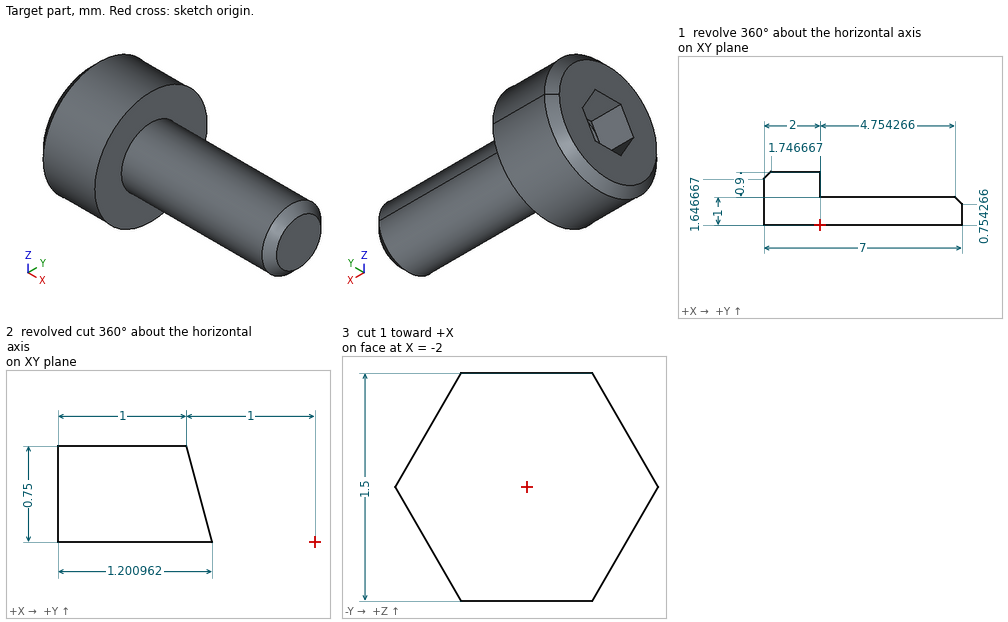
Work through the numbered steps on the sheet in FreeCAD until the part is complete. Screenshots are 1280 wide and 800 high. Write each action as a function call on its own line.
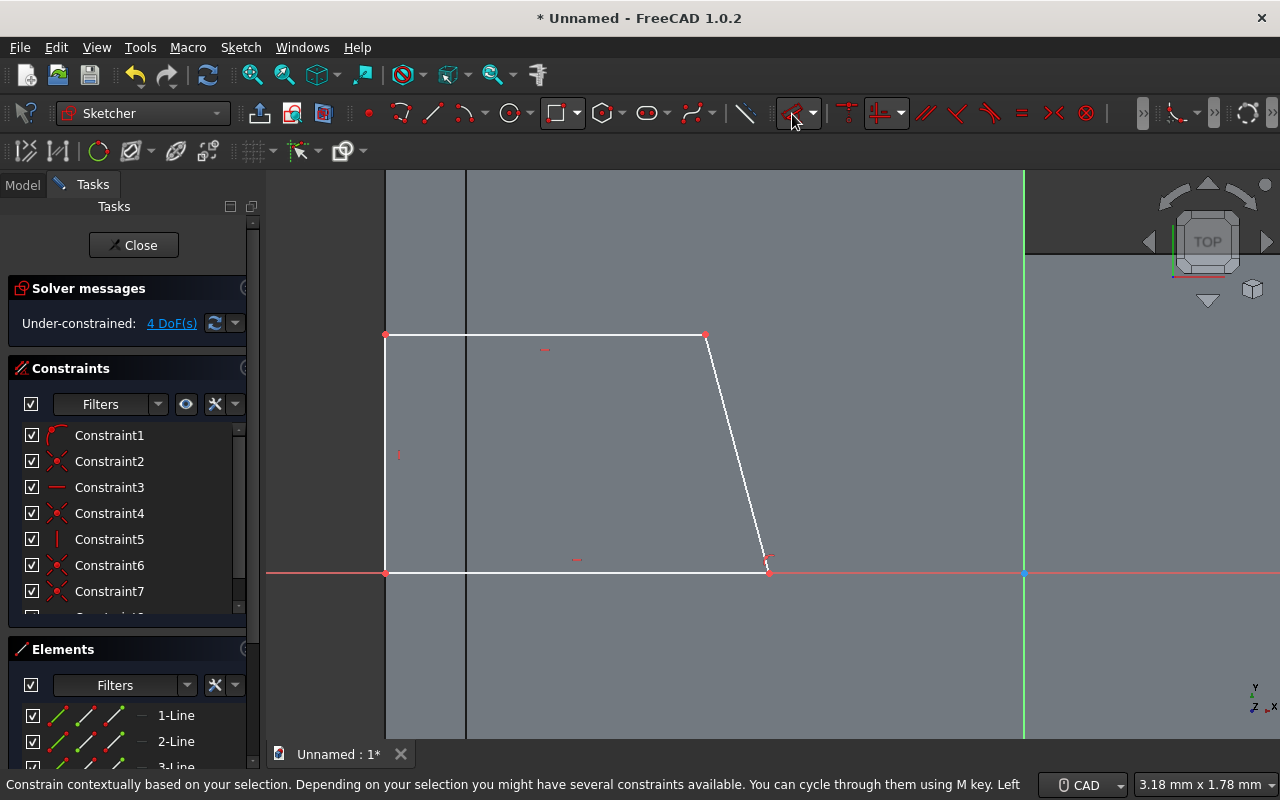
click(609, 335)
click(545, 301)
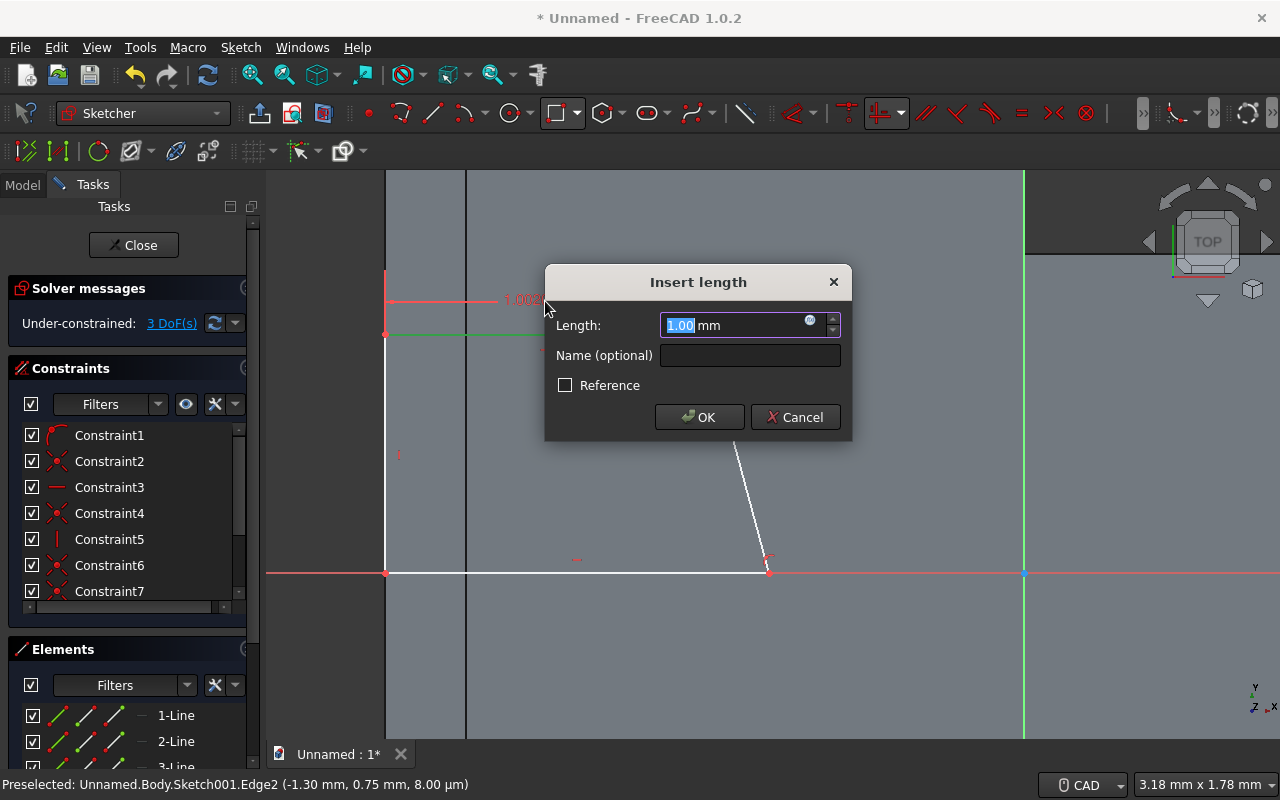
text(1)
key(Return)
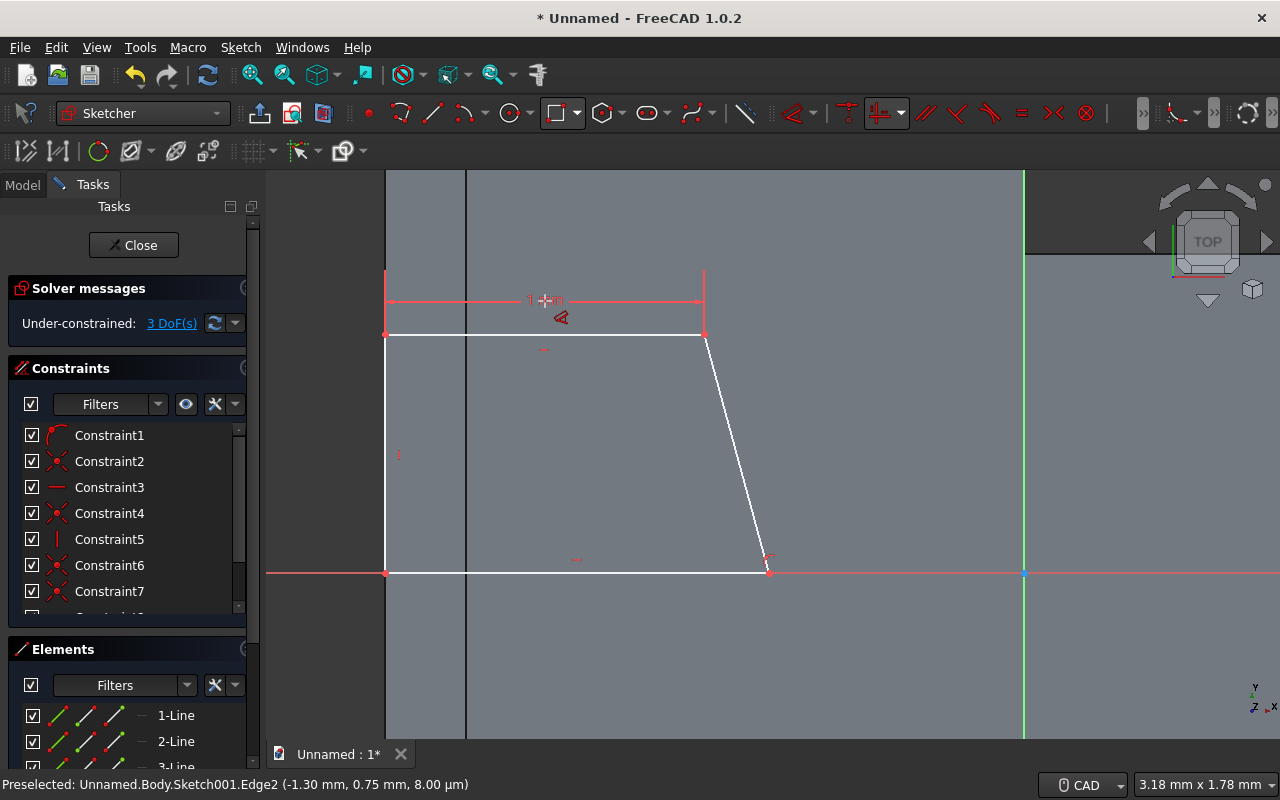
click(704, 335)
click(864, 607)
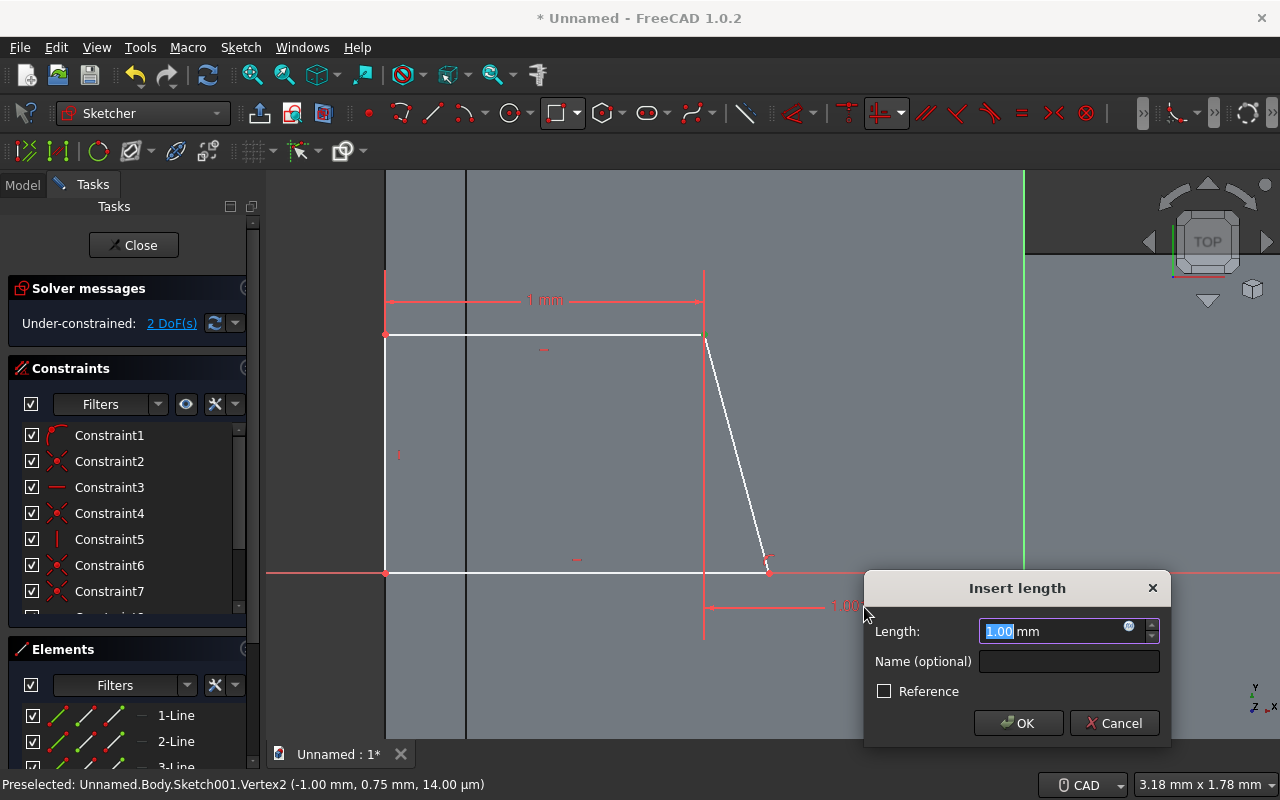
text(1)
key(Return)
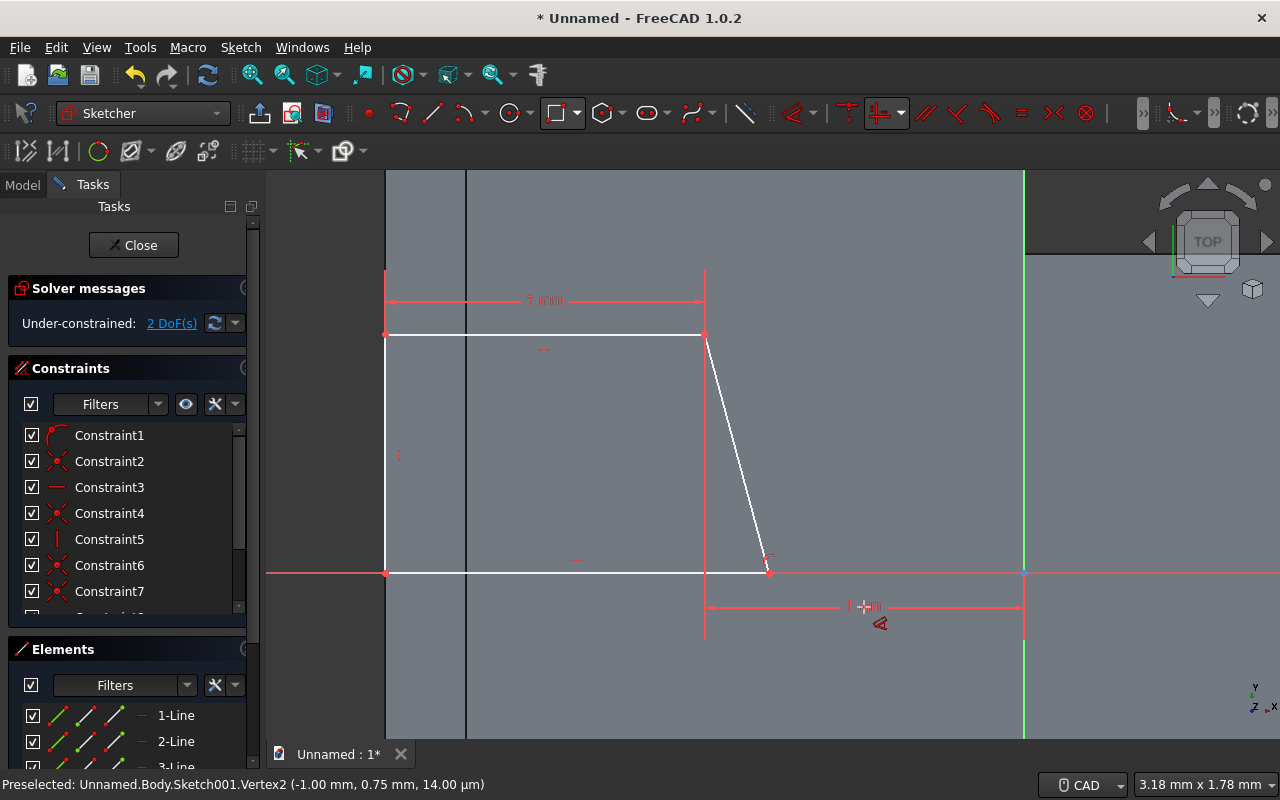
click(385, 406)
click(351, 454)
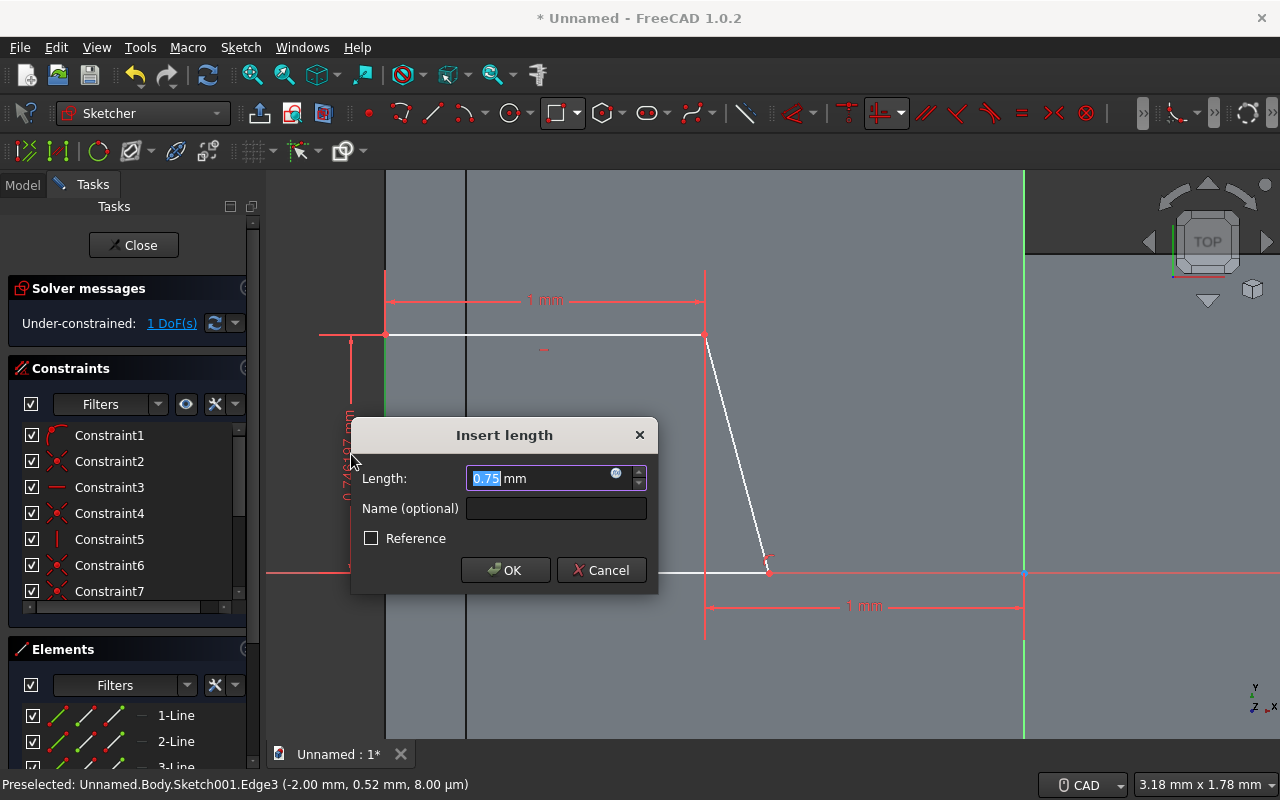
text(0.75)
key(Return)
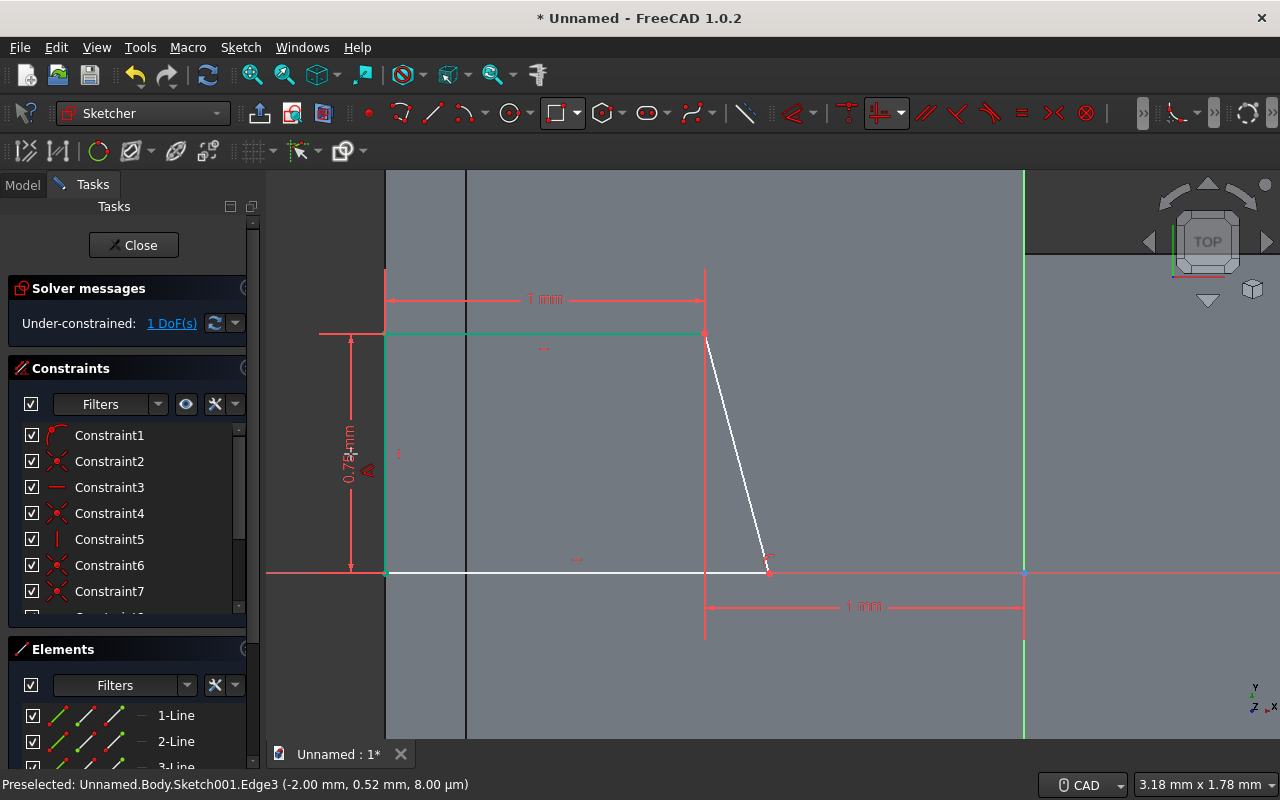
click(500, 573)
click(577, 607)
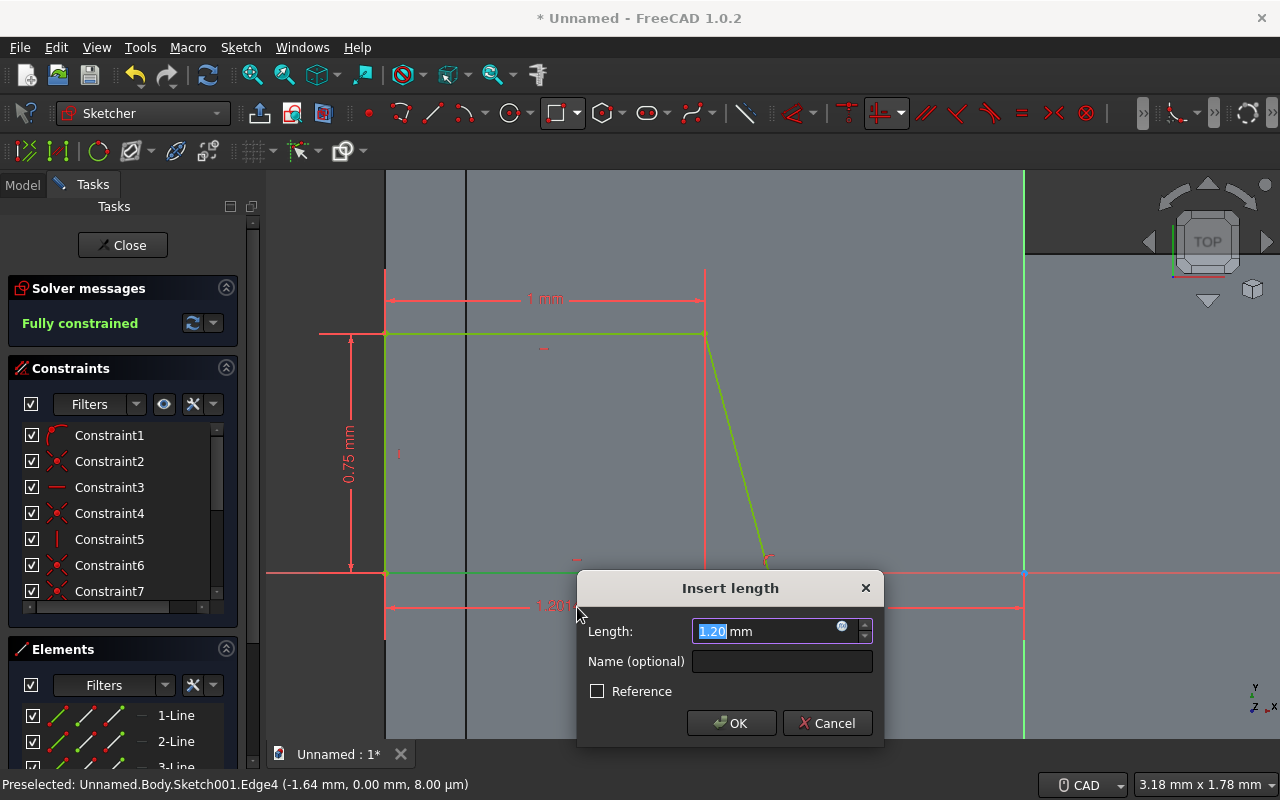
text(1.200962)
key(Return)
key(Escape)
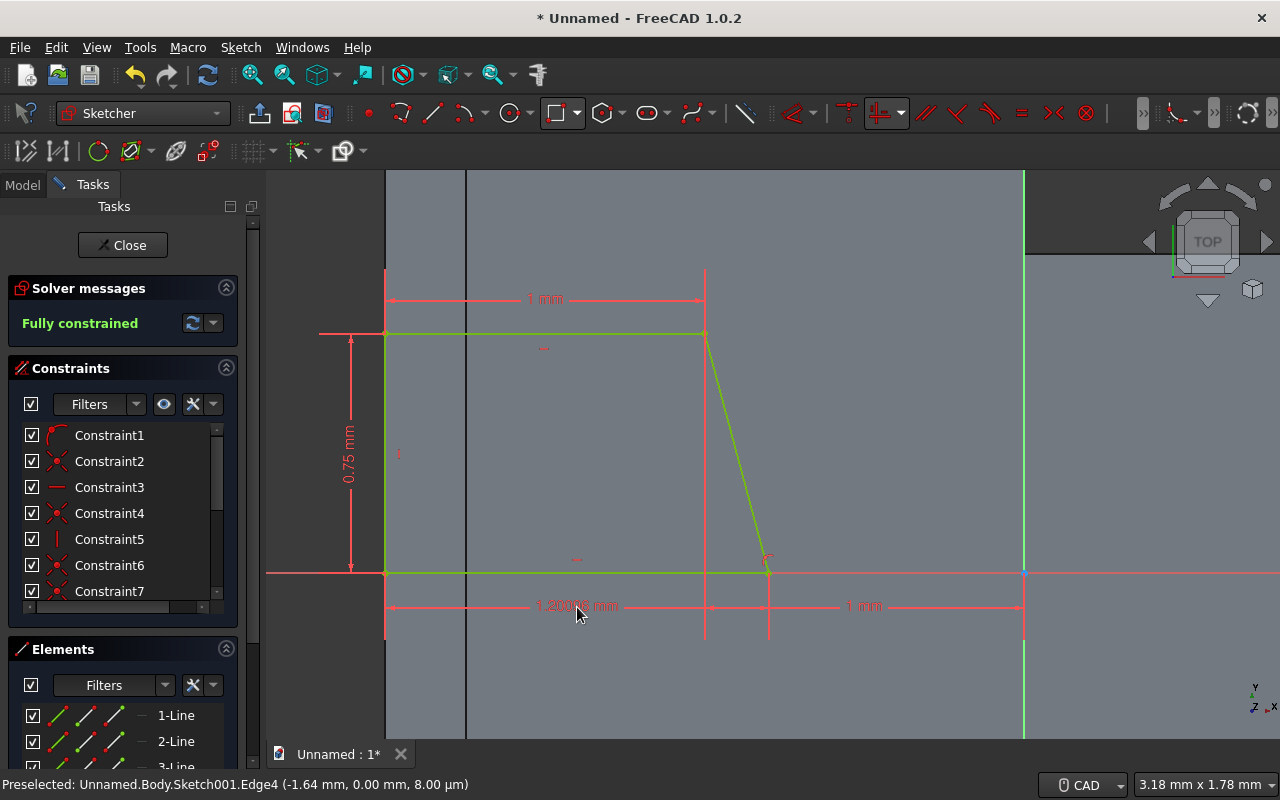
click(123, 245)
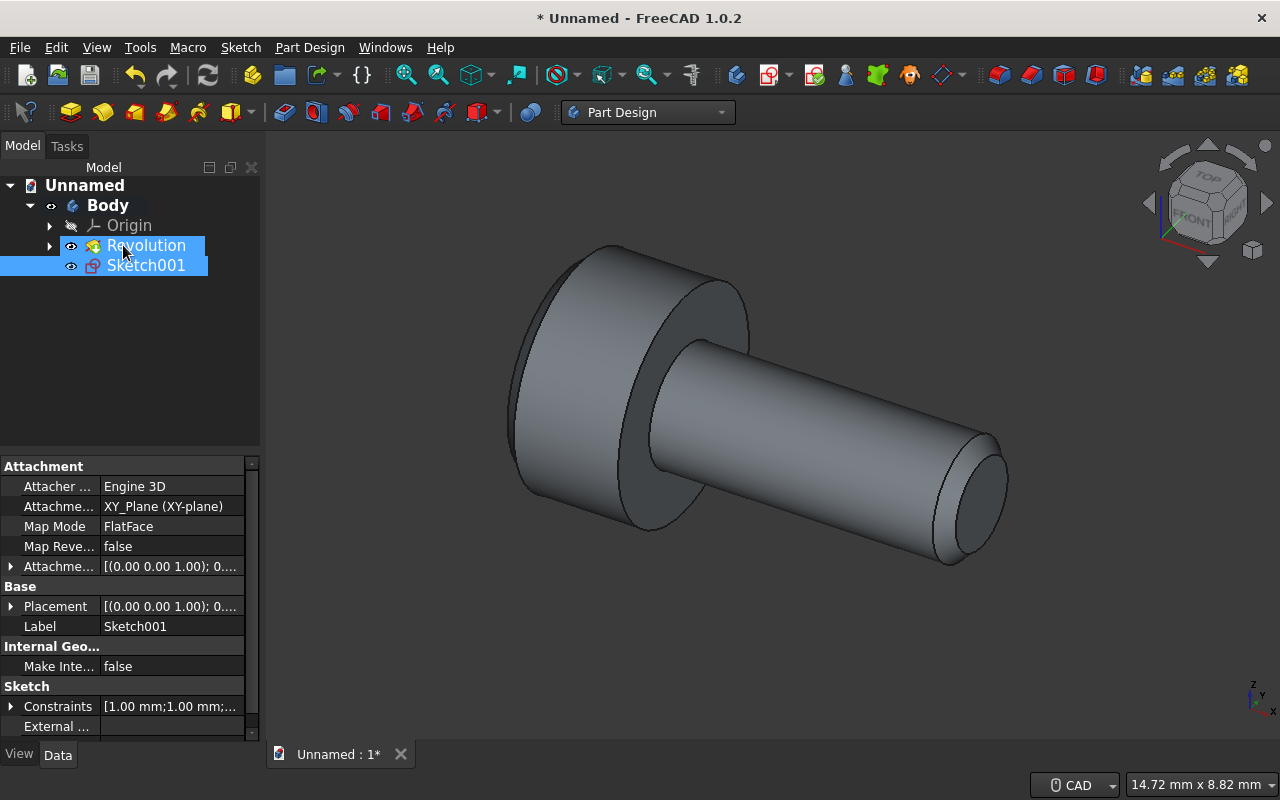
click(350, 112)